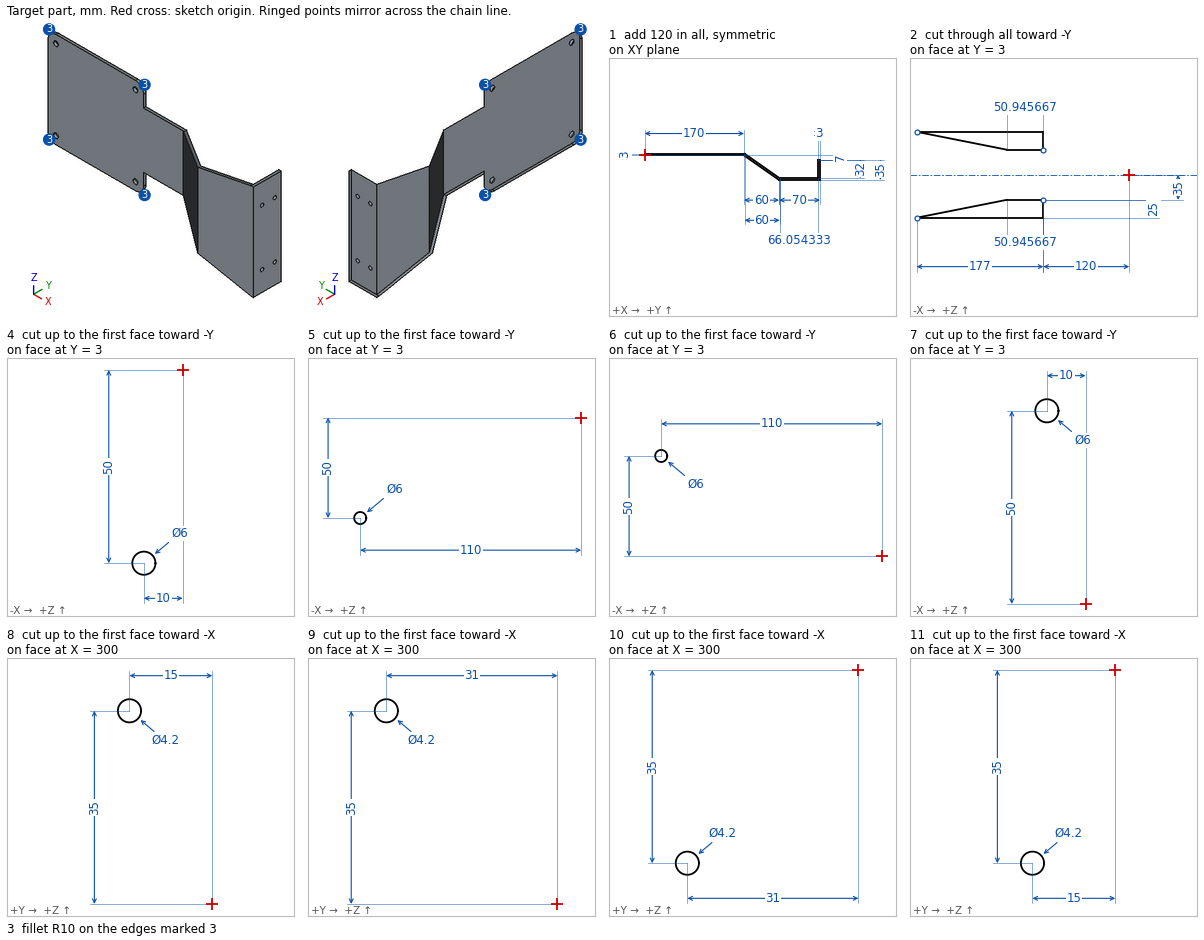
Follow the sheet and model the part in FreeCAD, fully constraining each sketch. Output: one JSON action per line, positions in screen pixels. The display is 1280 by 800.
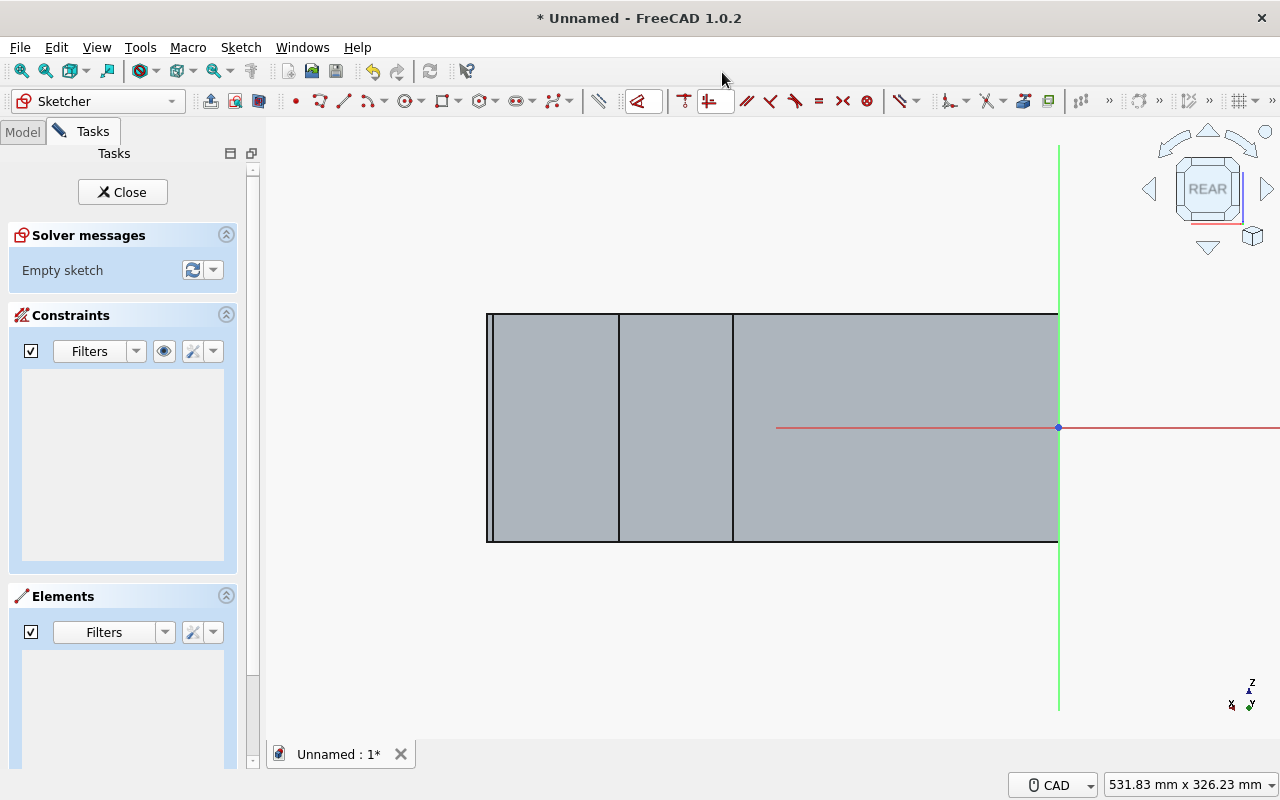
{"action": "left_click", "coordinate": [320, 102]}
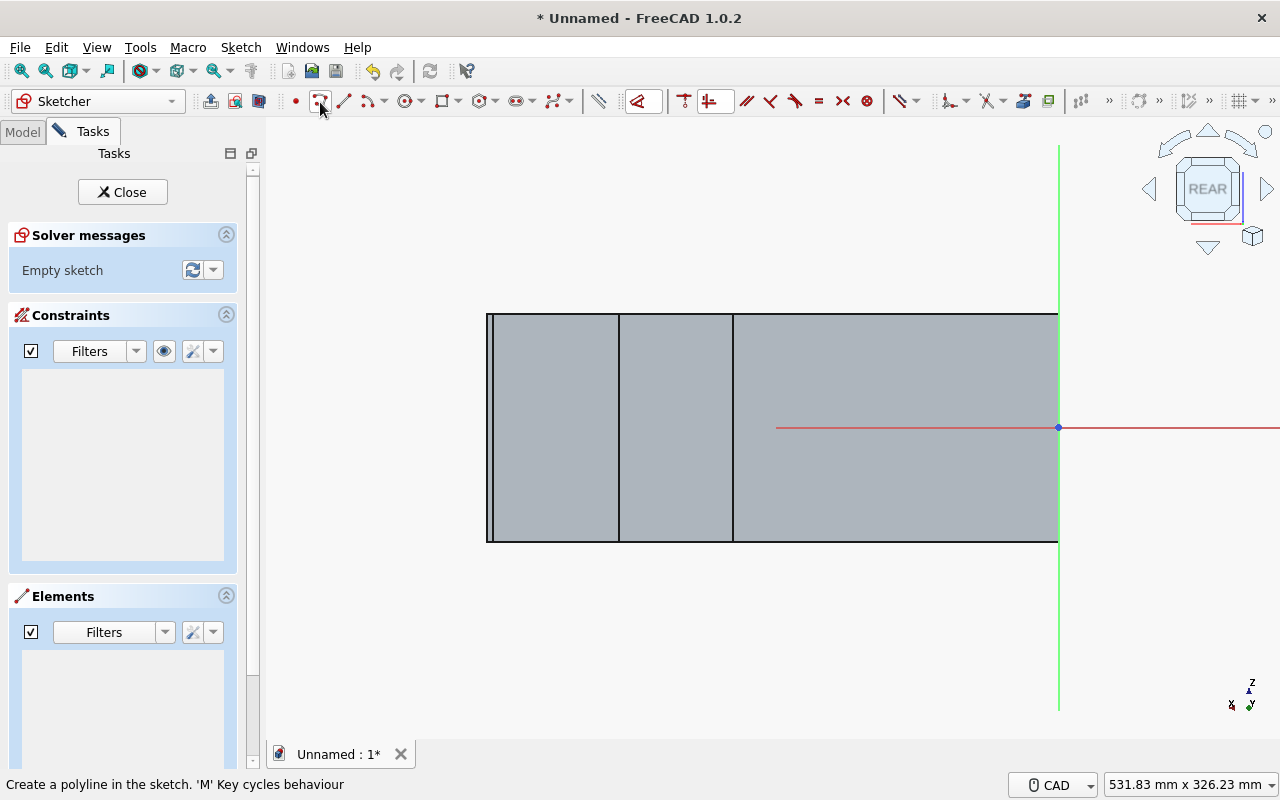
{"action": "left_click", "coordinate": [830, 495]}
{"action": "left_click", "coordinate": [733, 495]}
{"action": "left_click", "coordinate": [493, 542]}
{"action": "left_click", "coordinate": [830, 542]}
{"action": "left_click", "coordinate": [830, 496]}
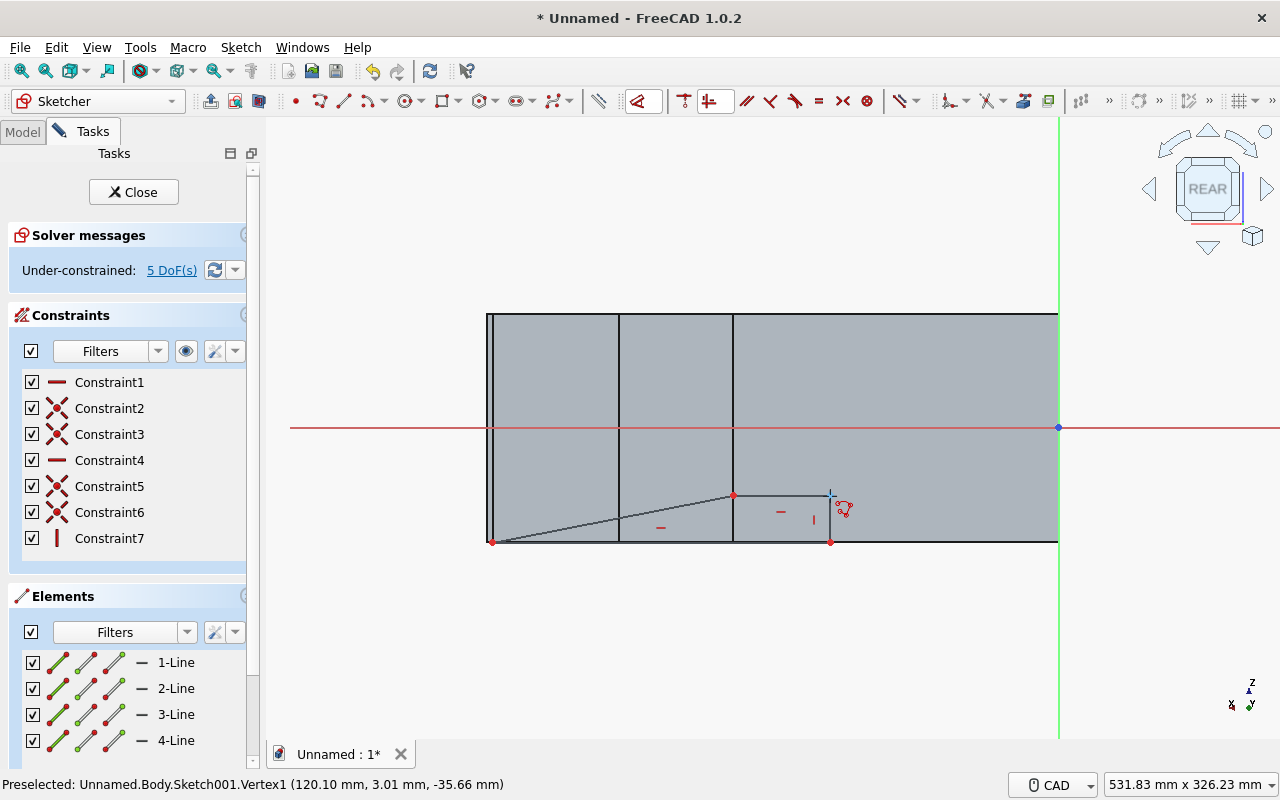
{"action": "left_click", "coordinate": [830, 361]}
{"action": "left_click", "coordinate": [830, 314]}
{"action": "left_click", "coordinate": [493, 314]}
{"action": "left_click", "coordinate": [733, 361]}
{"action": "left_click", "coordinate": [830, 362]}
{"action": "key", "text": "Escape"}
{"action": "key", "text": "Escape"}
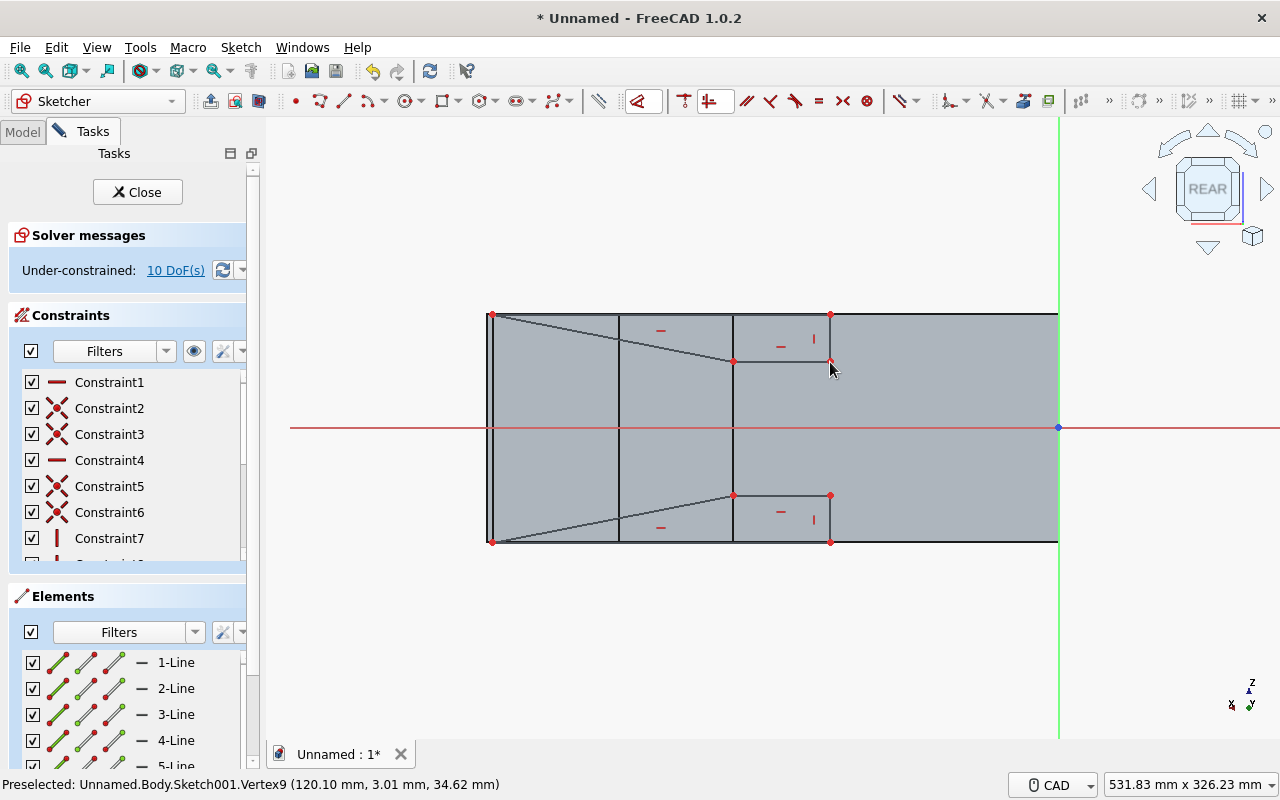
{"action": "left_click", "coordinate": [830, 496]}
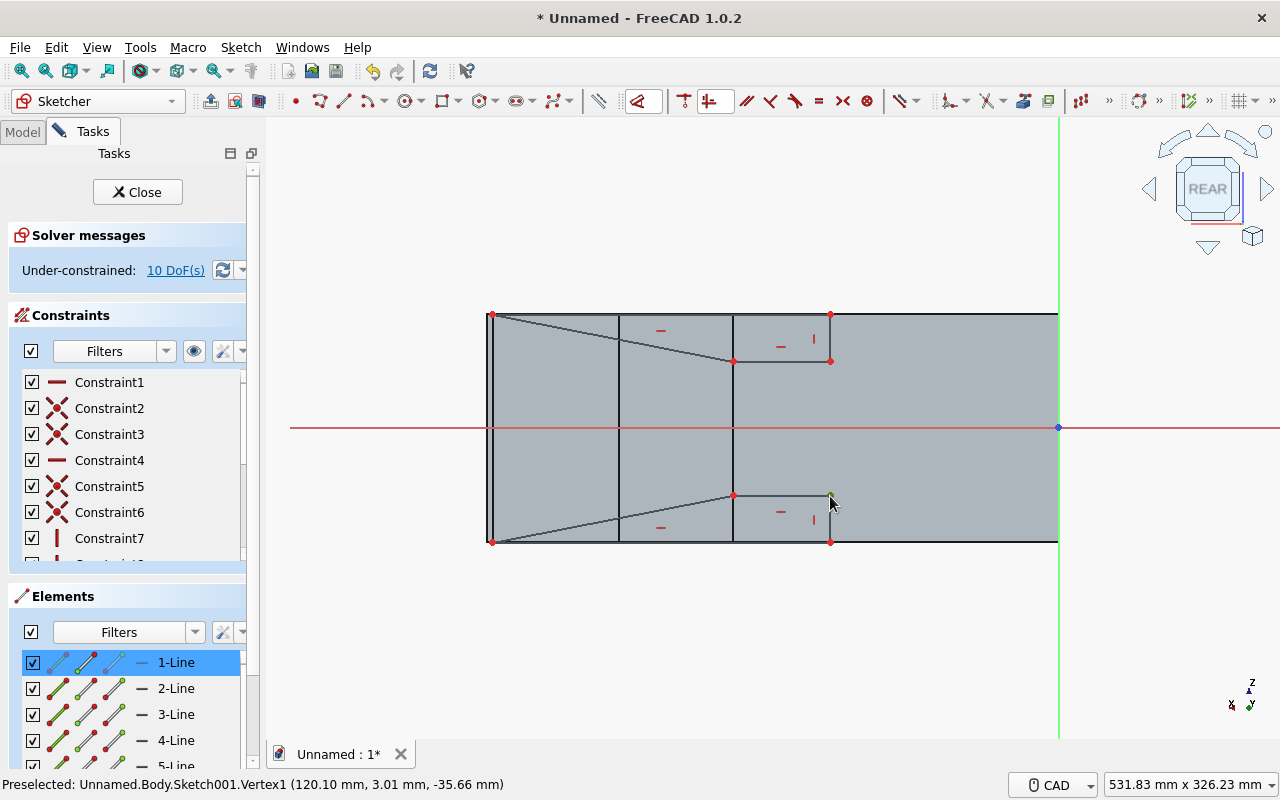
{"action": "left_click", "coordinate": [830, 362]}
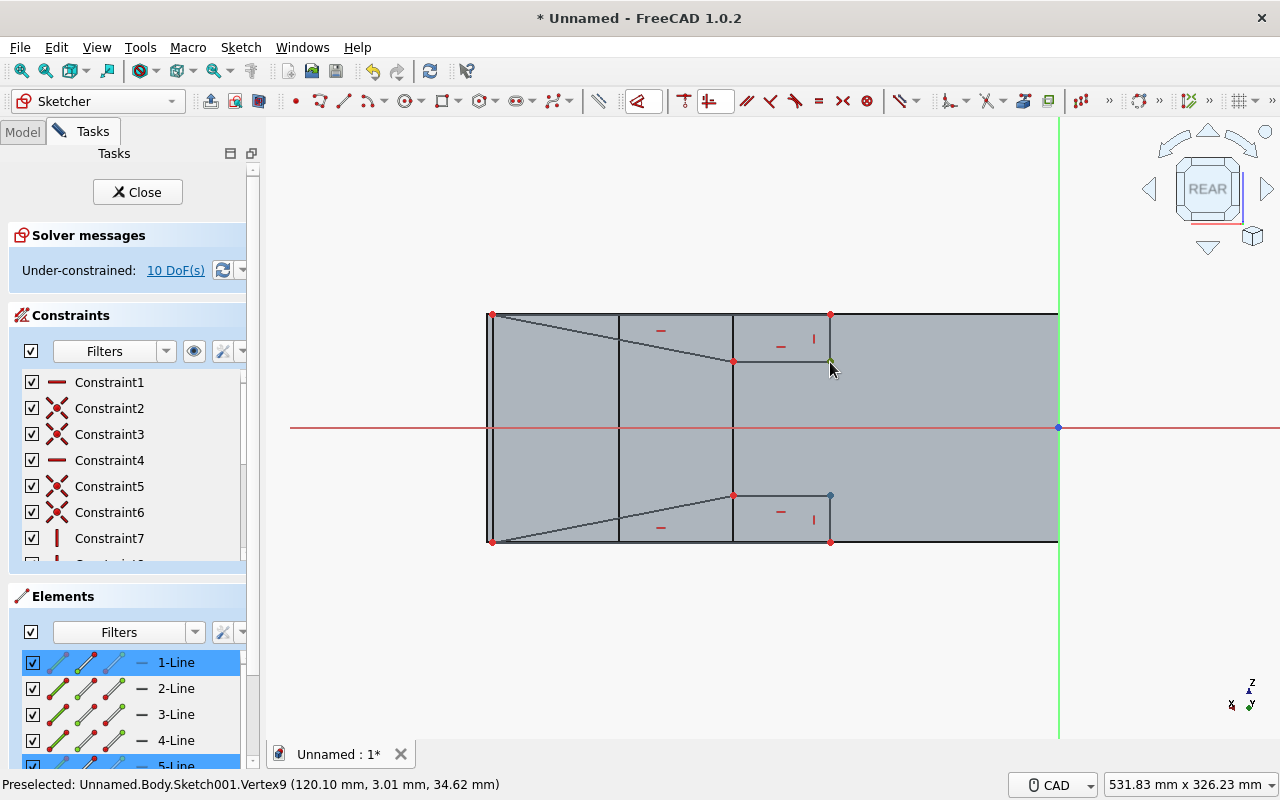
{"action": "left_click", "coordinate": [353, 428]}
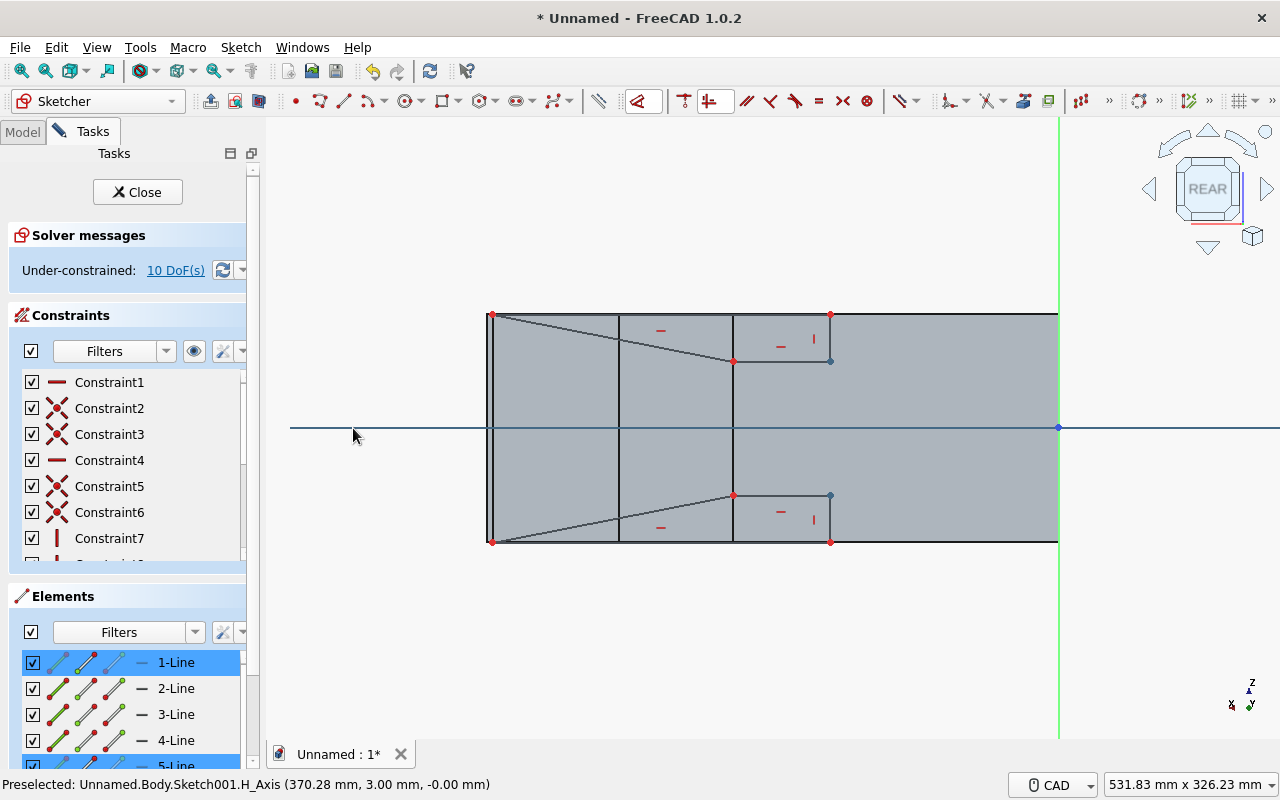
{"action": "left_click", "coordinate": [844, 102]}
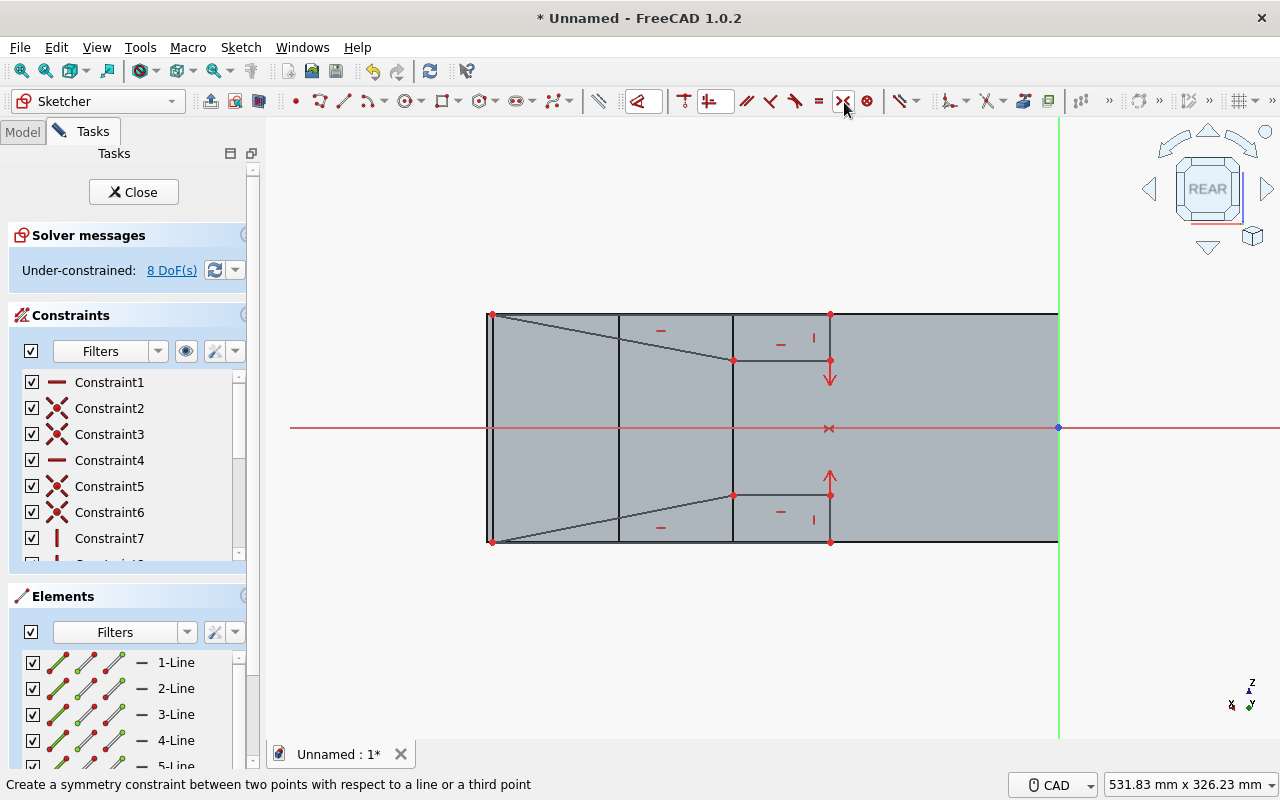
{"action": "left_click", "coordinate": [493, 543]}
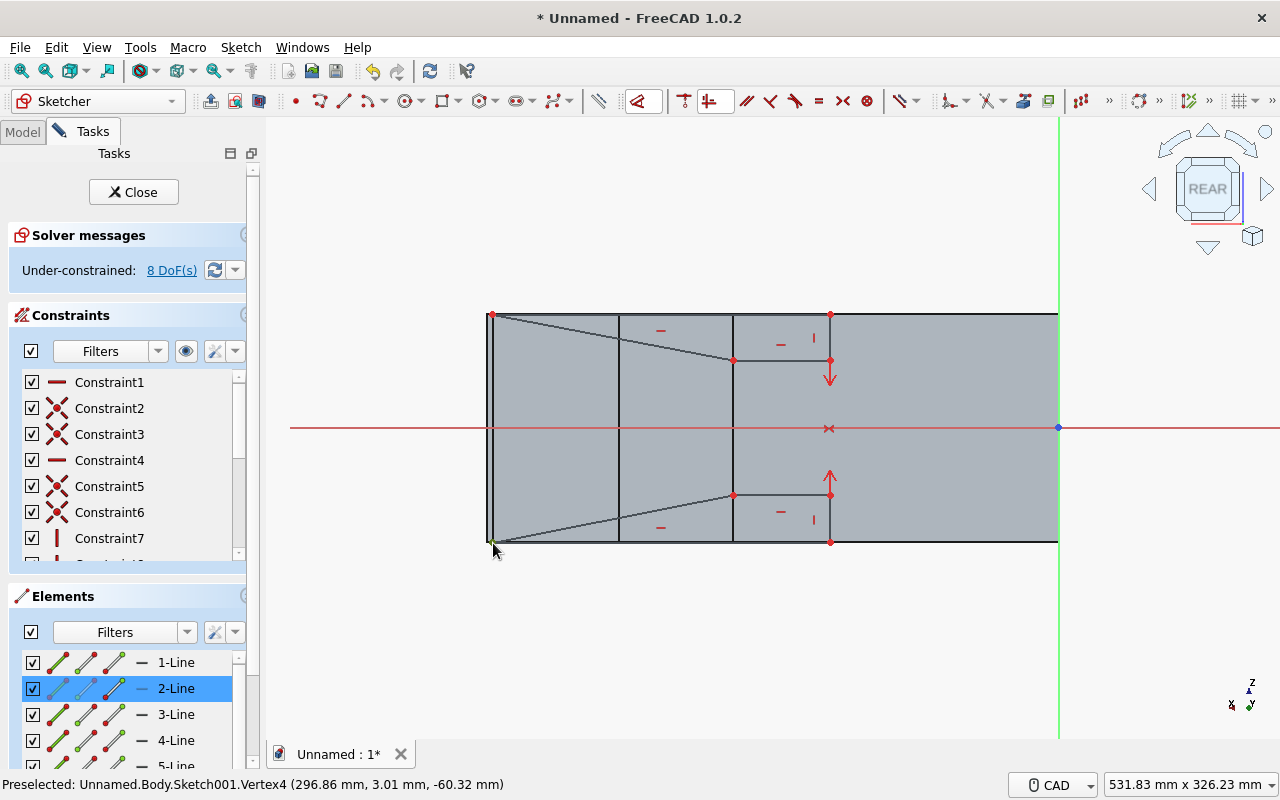
{"action": "left_click", "coordinate": [493, 315]}